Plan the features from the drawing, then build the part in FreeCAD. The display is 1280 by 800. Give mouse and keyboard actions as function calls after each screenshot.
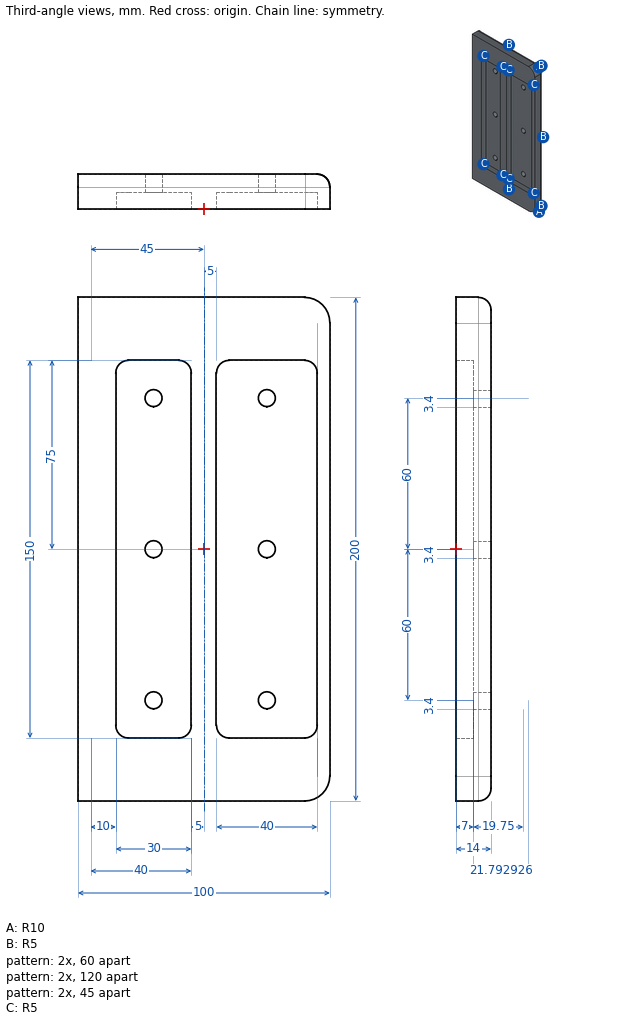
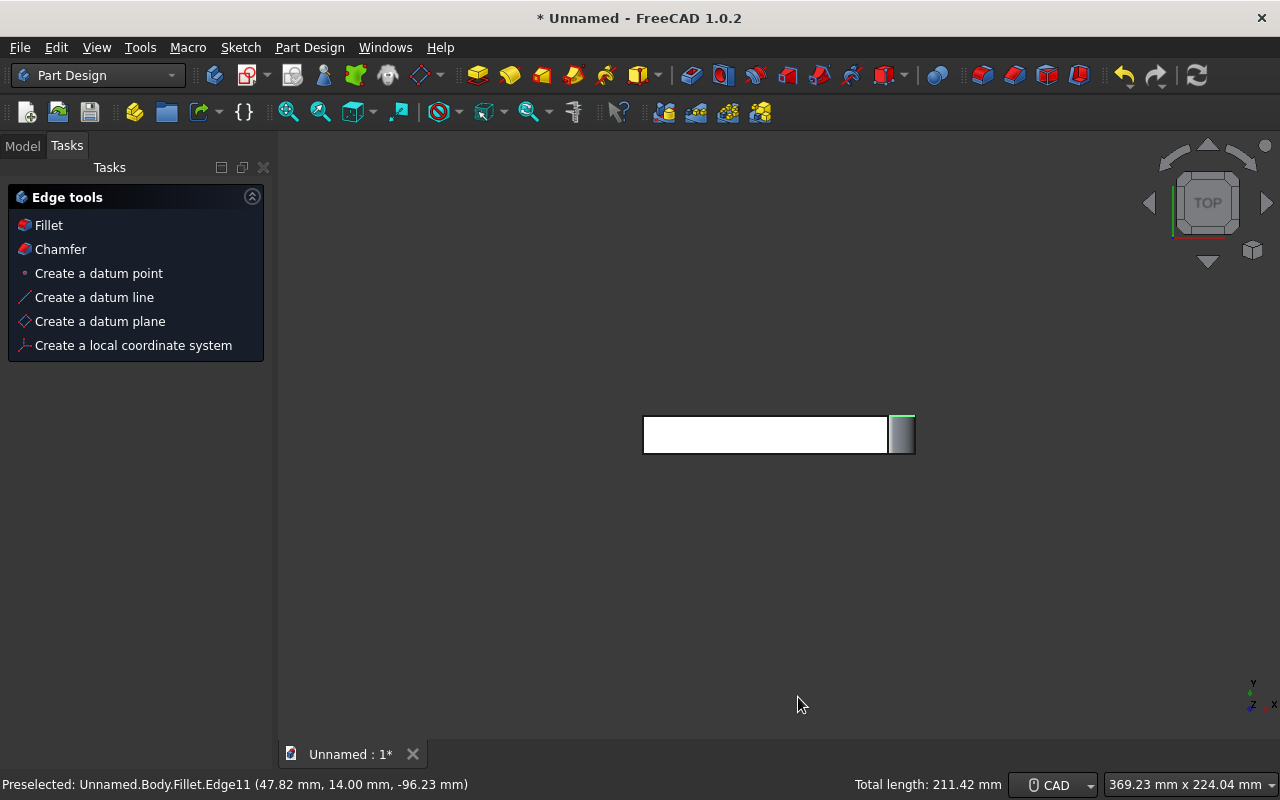
click(765, 415, ctrl)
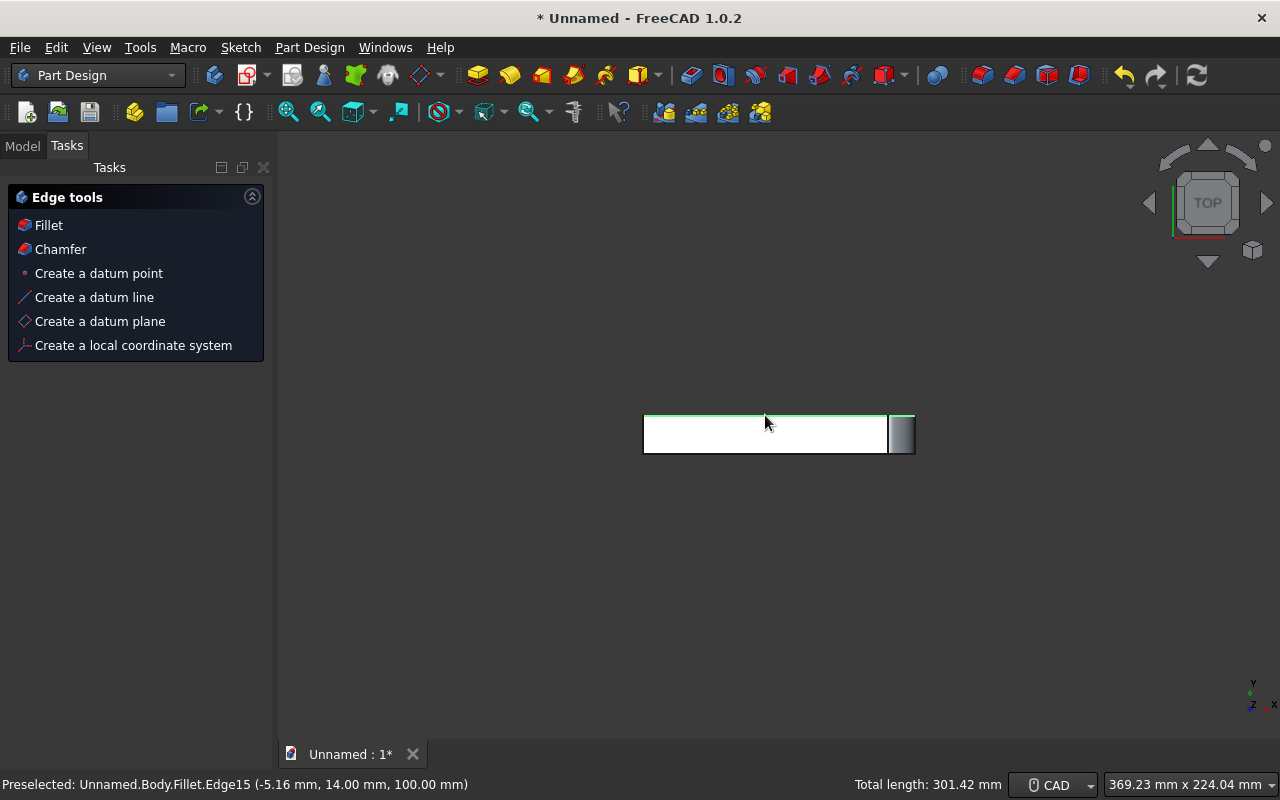
key(1)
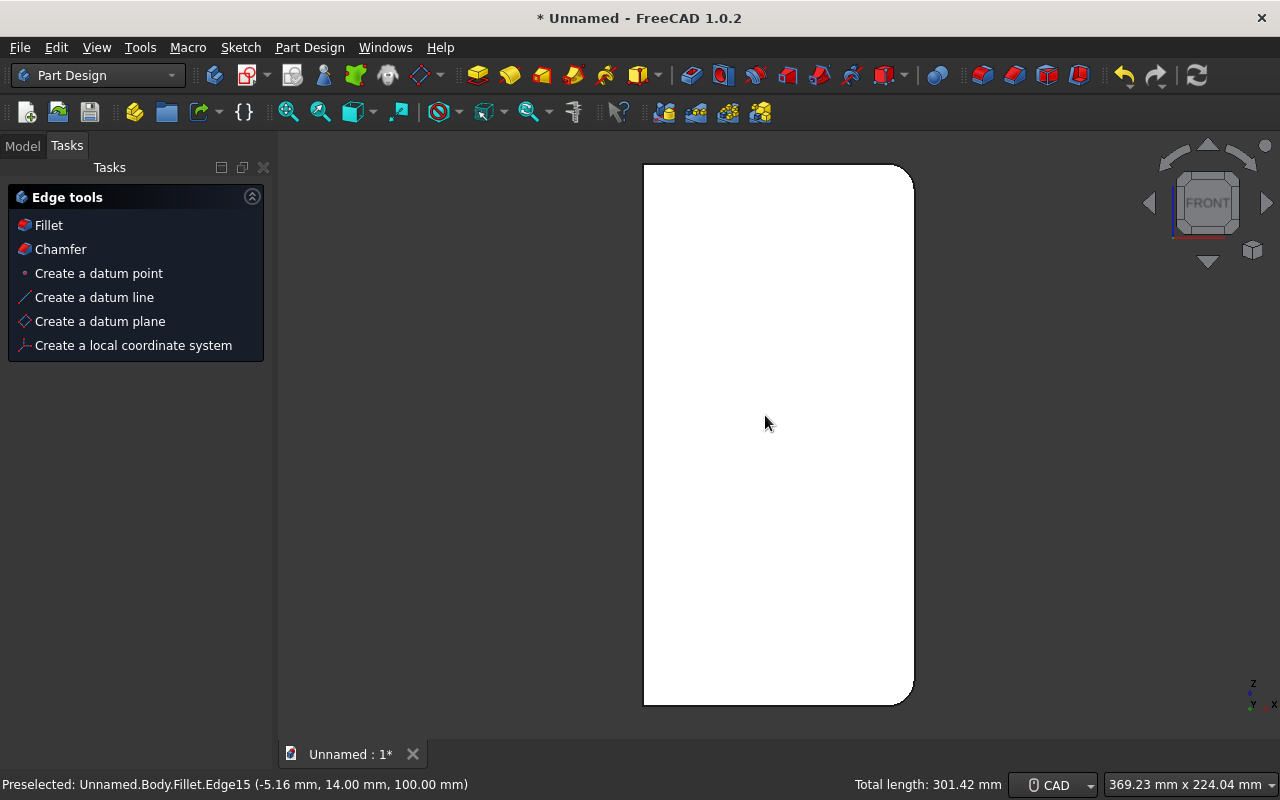
key(3)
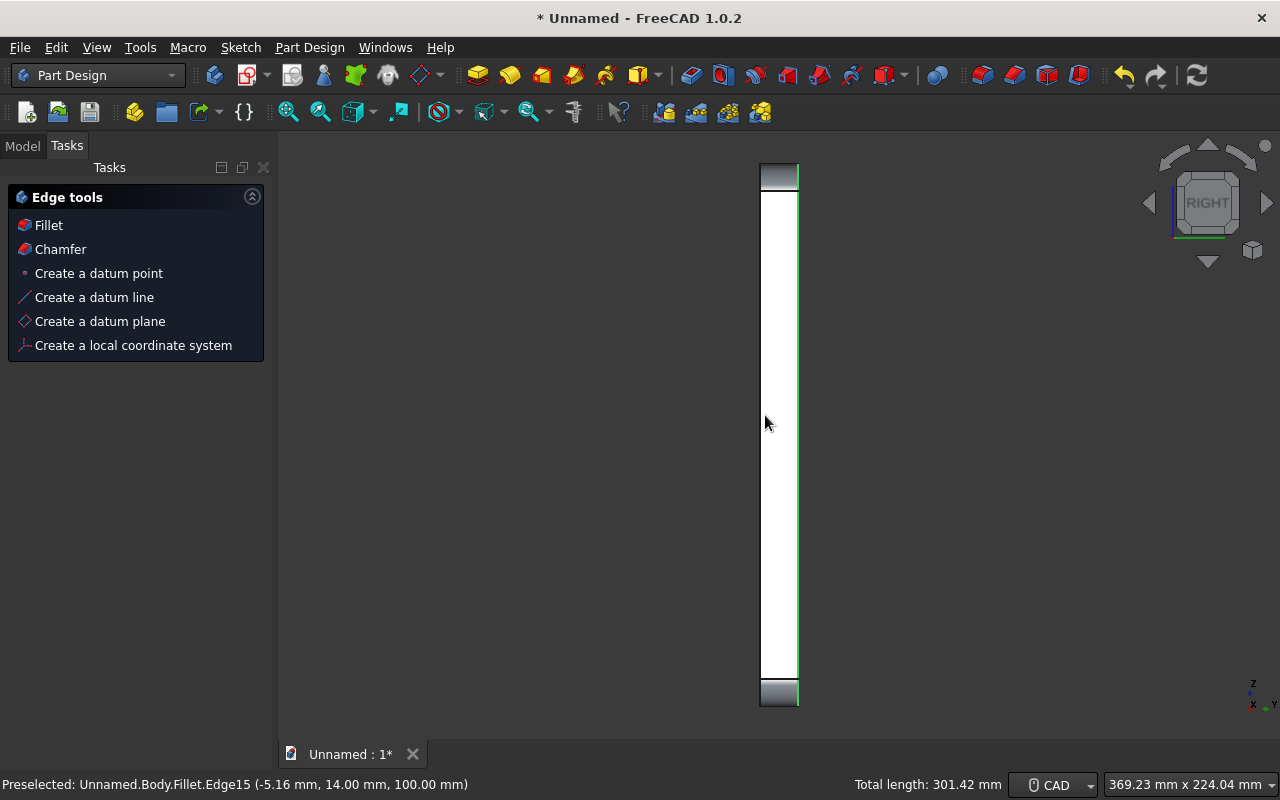
key(5)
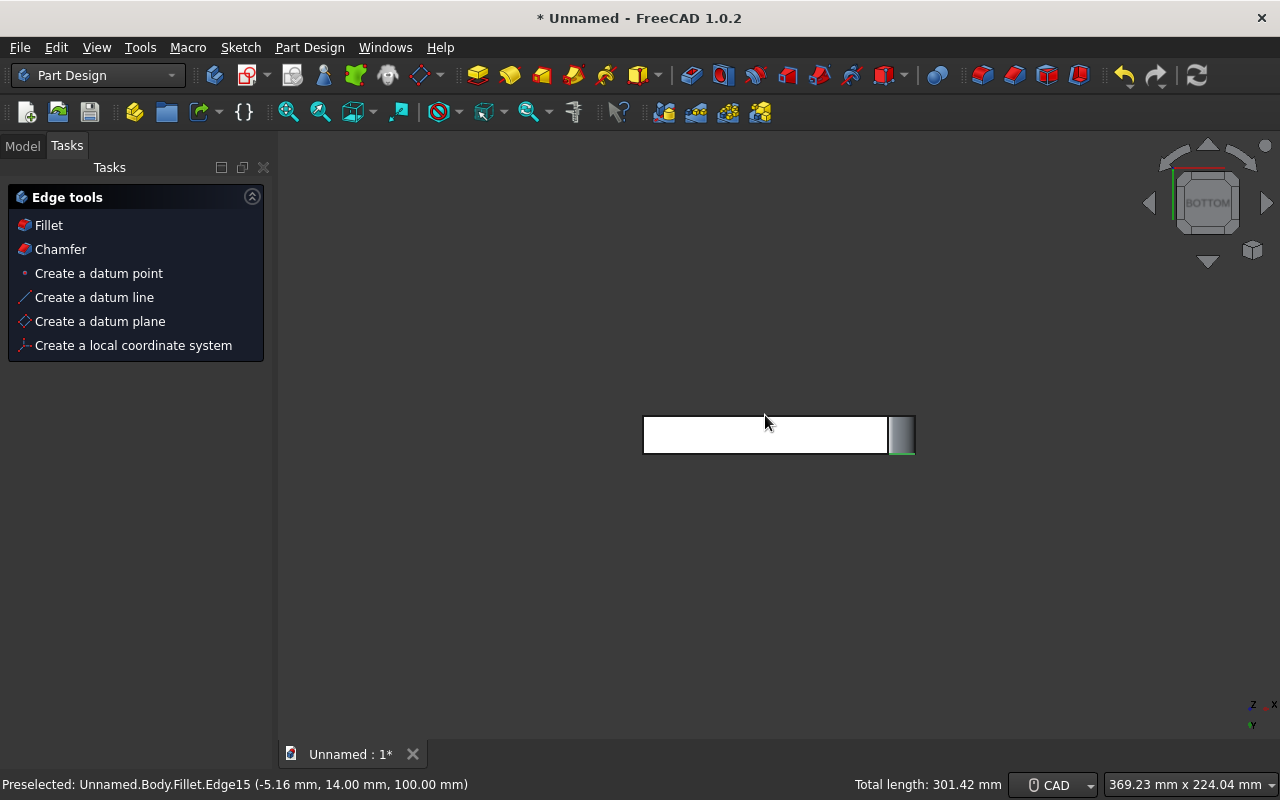
click(290, 112)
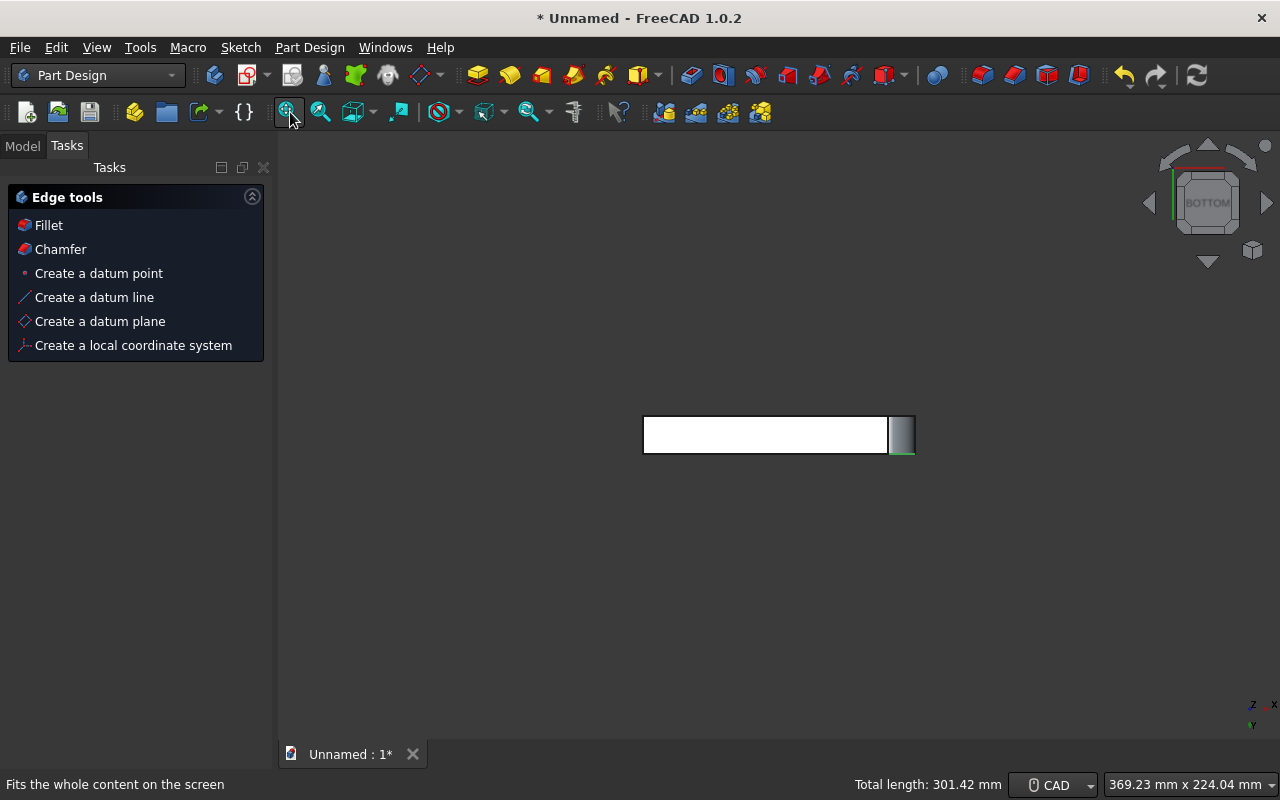
key(4)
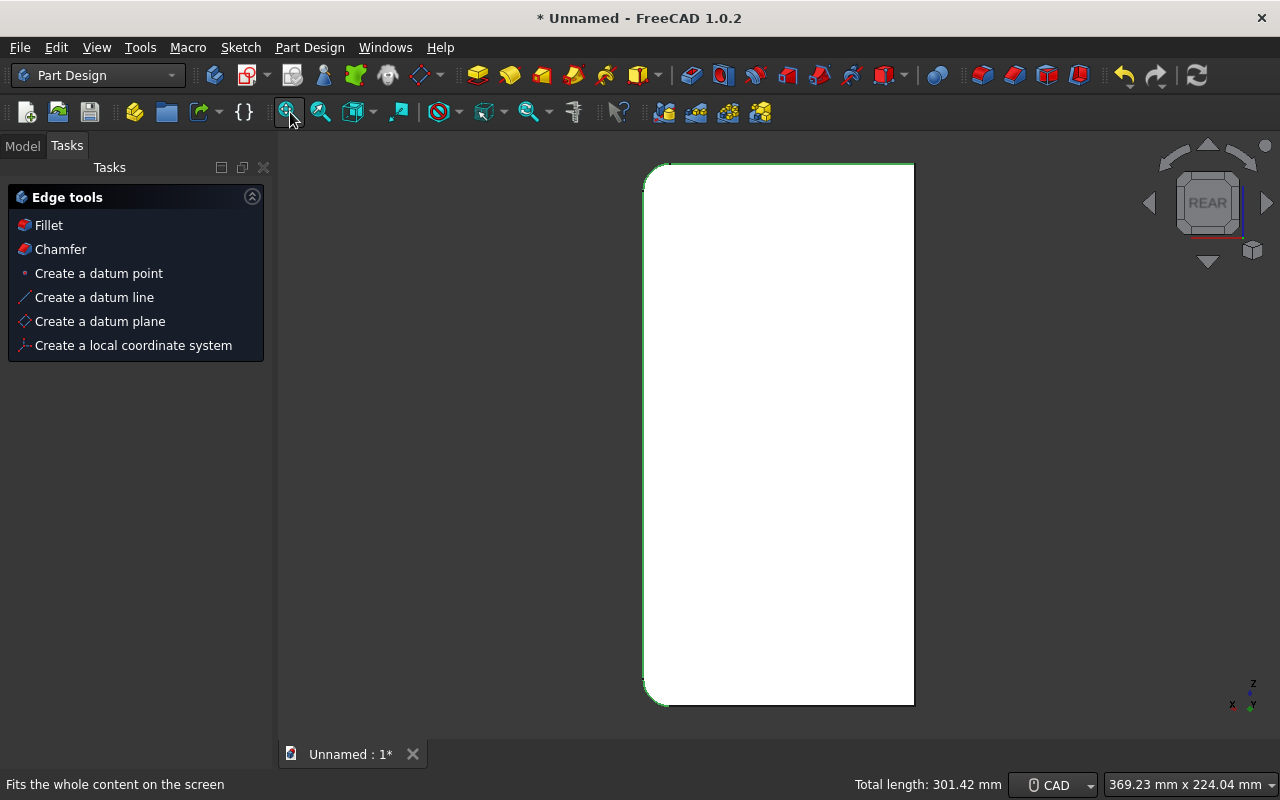
click(793, 705, ctrl)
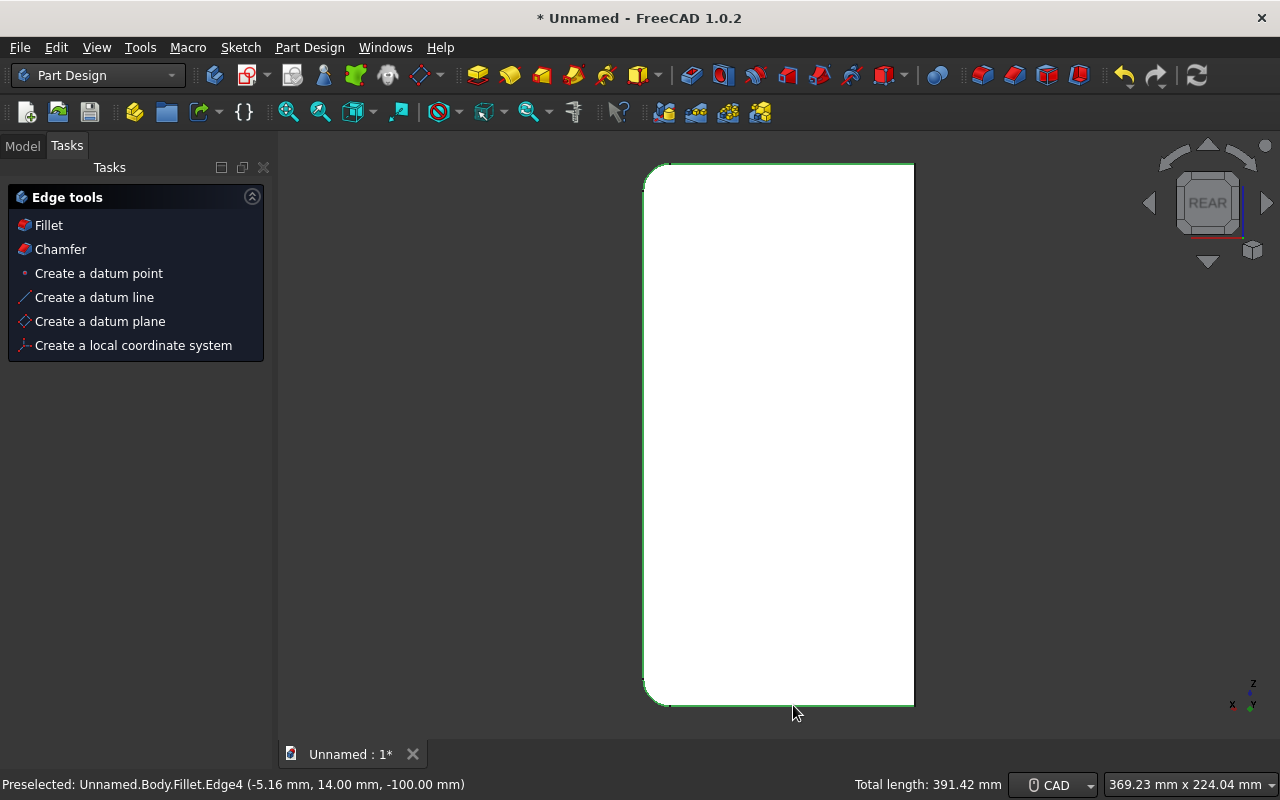
click(984, 76)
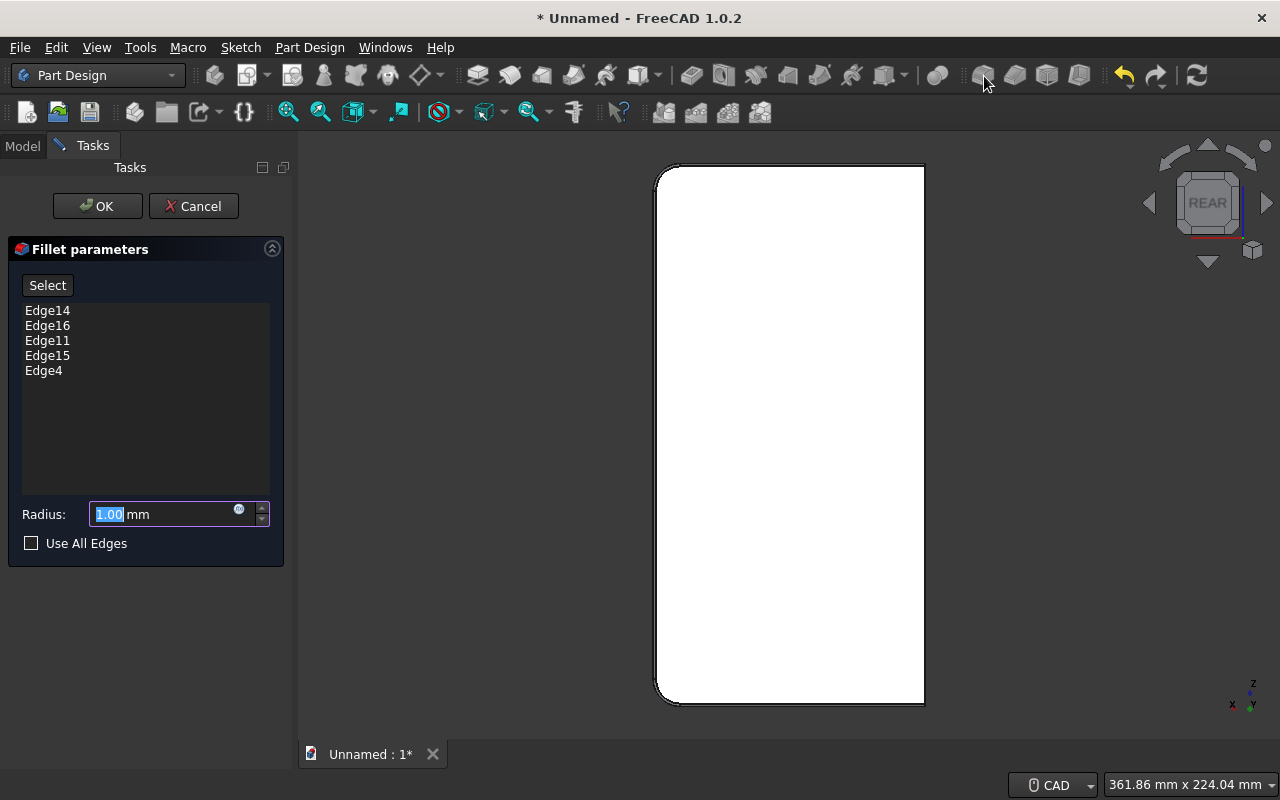
text(5)
key(Tab)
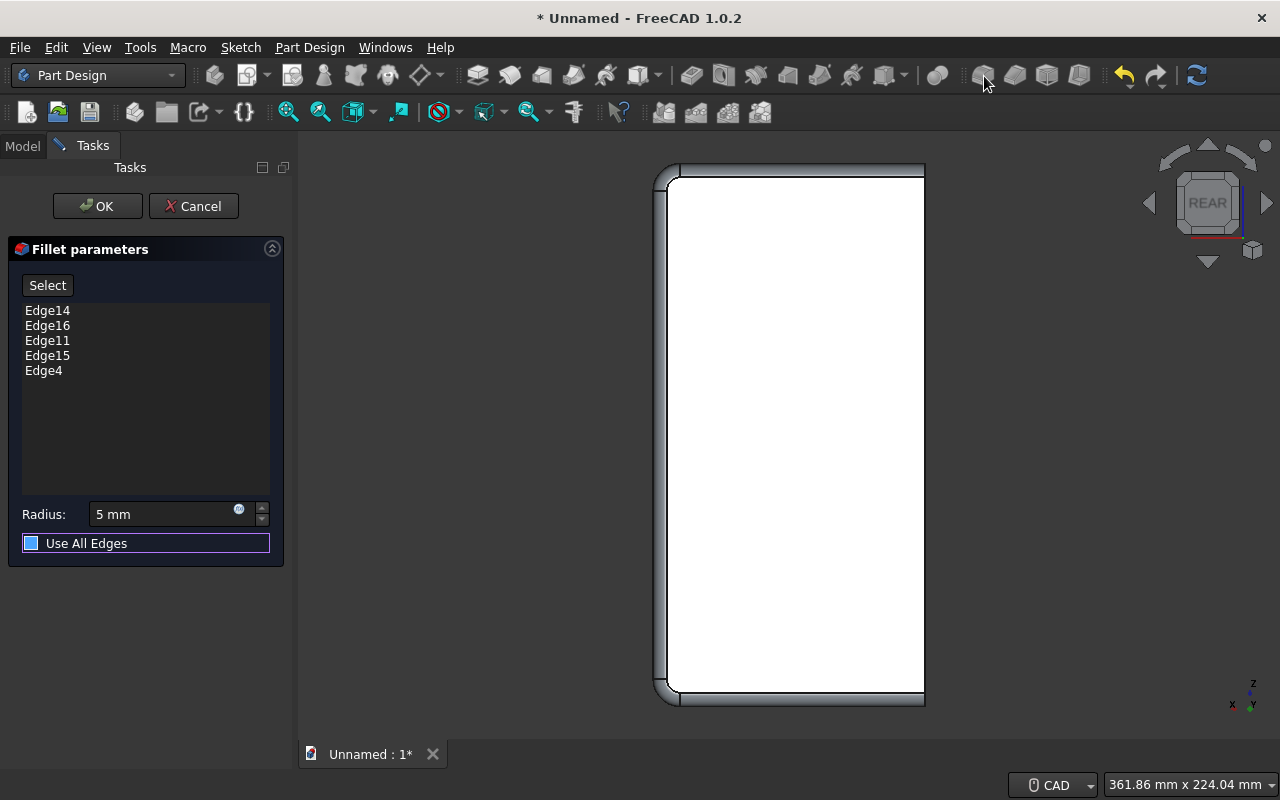
click(98, 206)